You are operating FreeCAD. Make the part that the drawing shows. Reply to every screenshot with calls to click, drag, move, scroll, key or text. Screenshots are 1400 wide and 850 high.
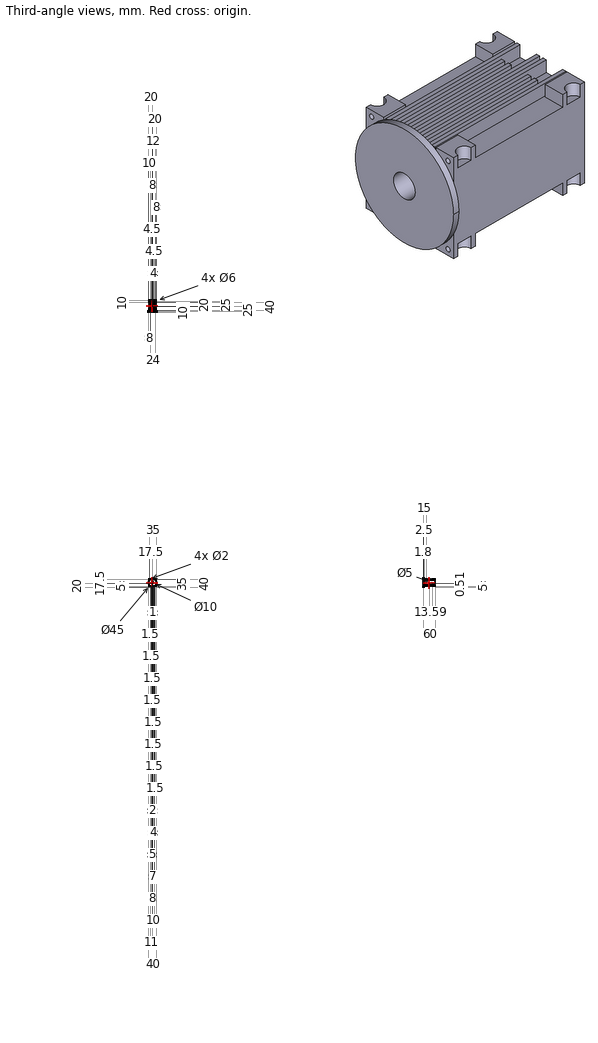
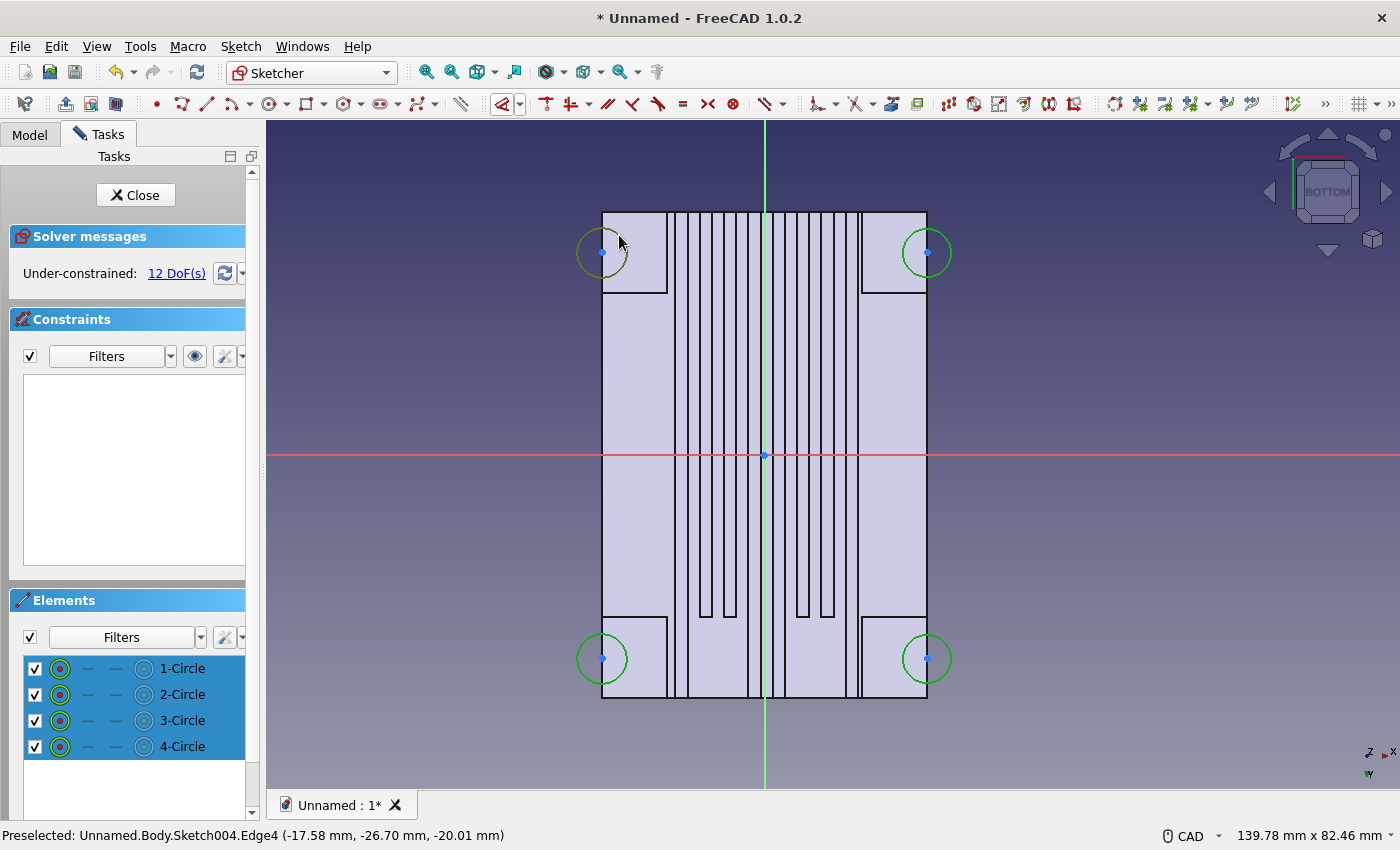
key(e)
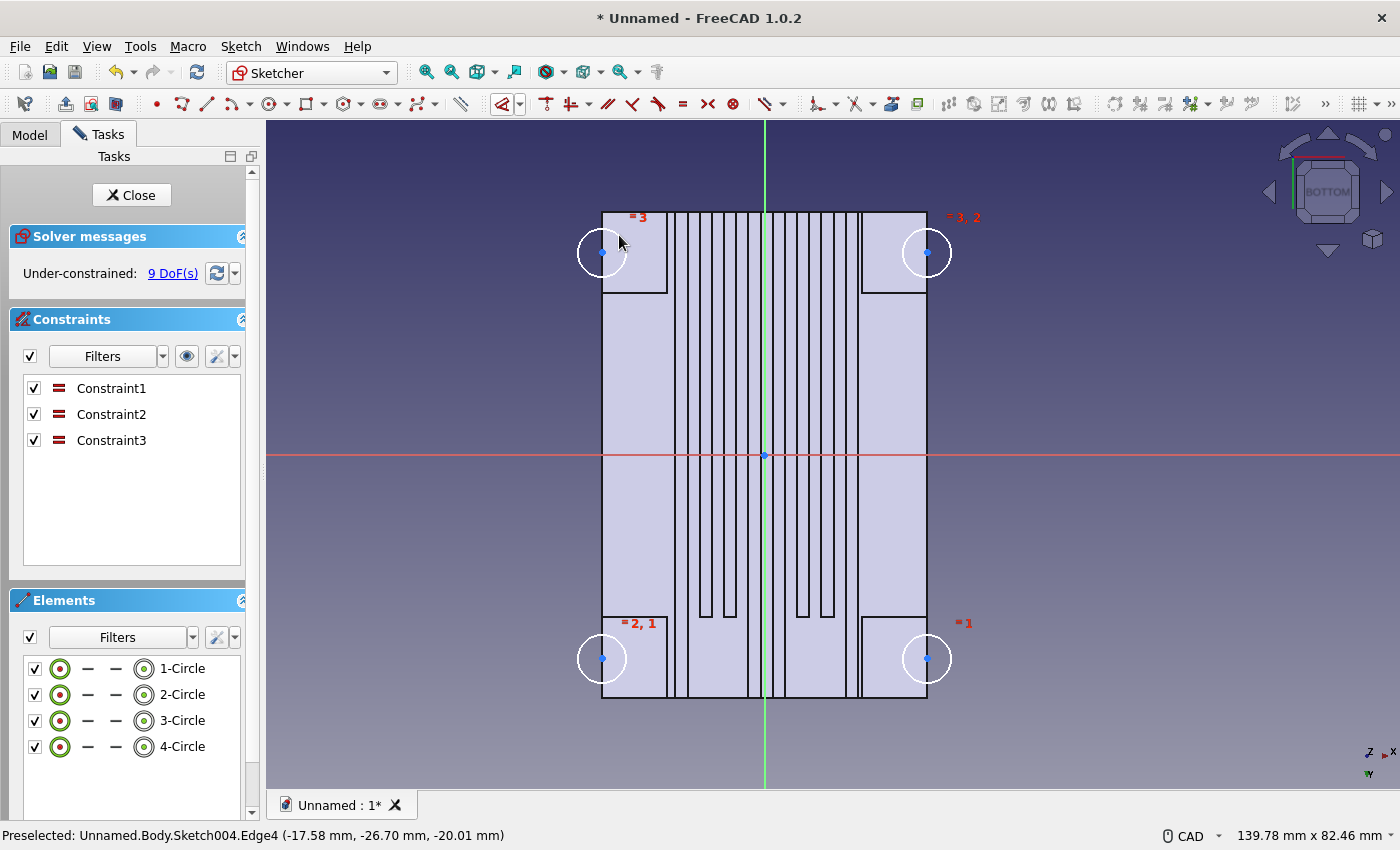
click(927, 659)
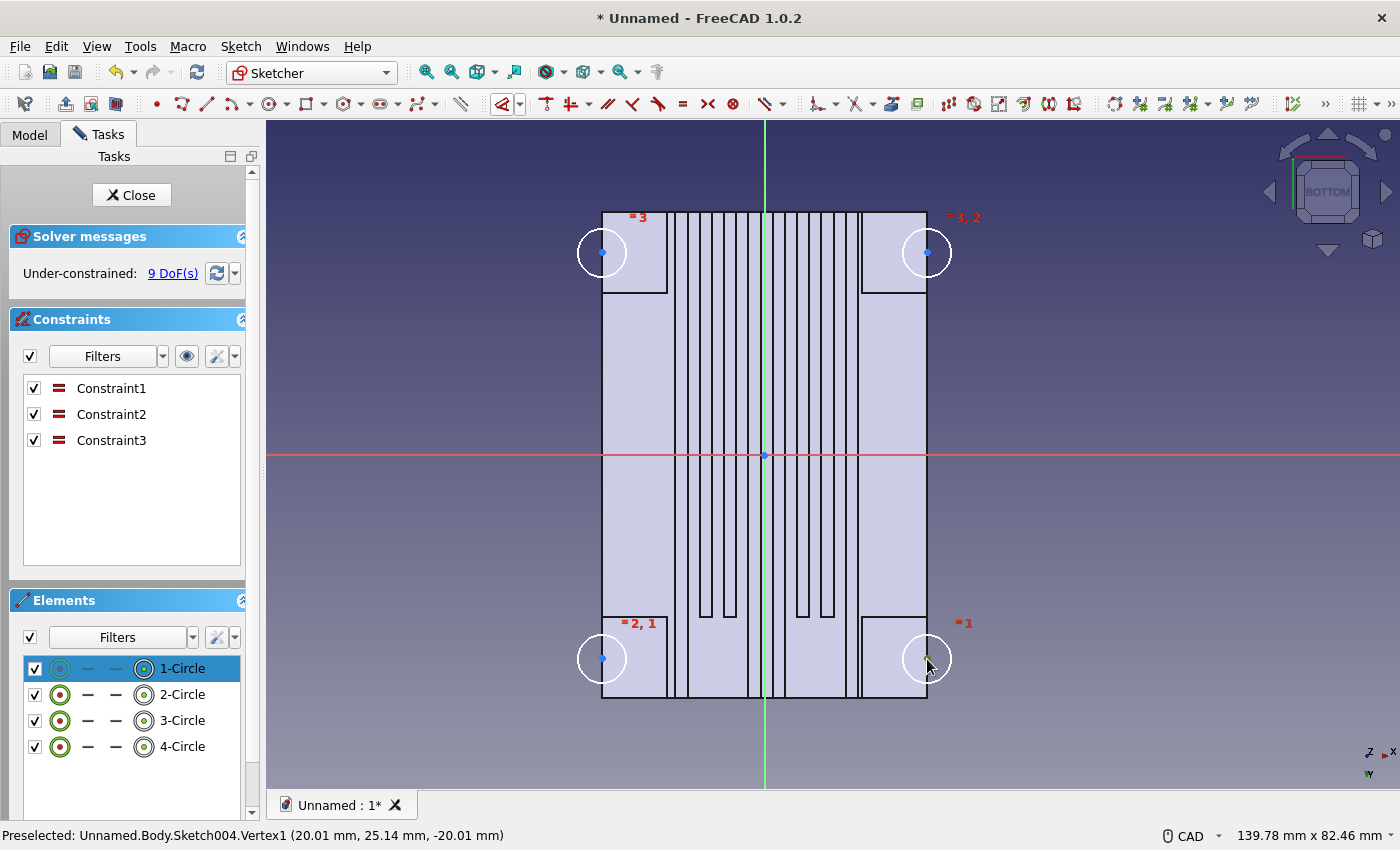
click(602, 659)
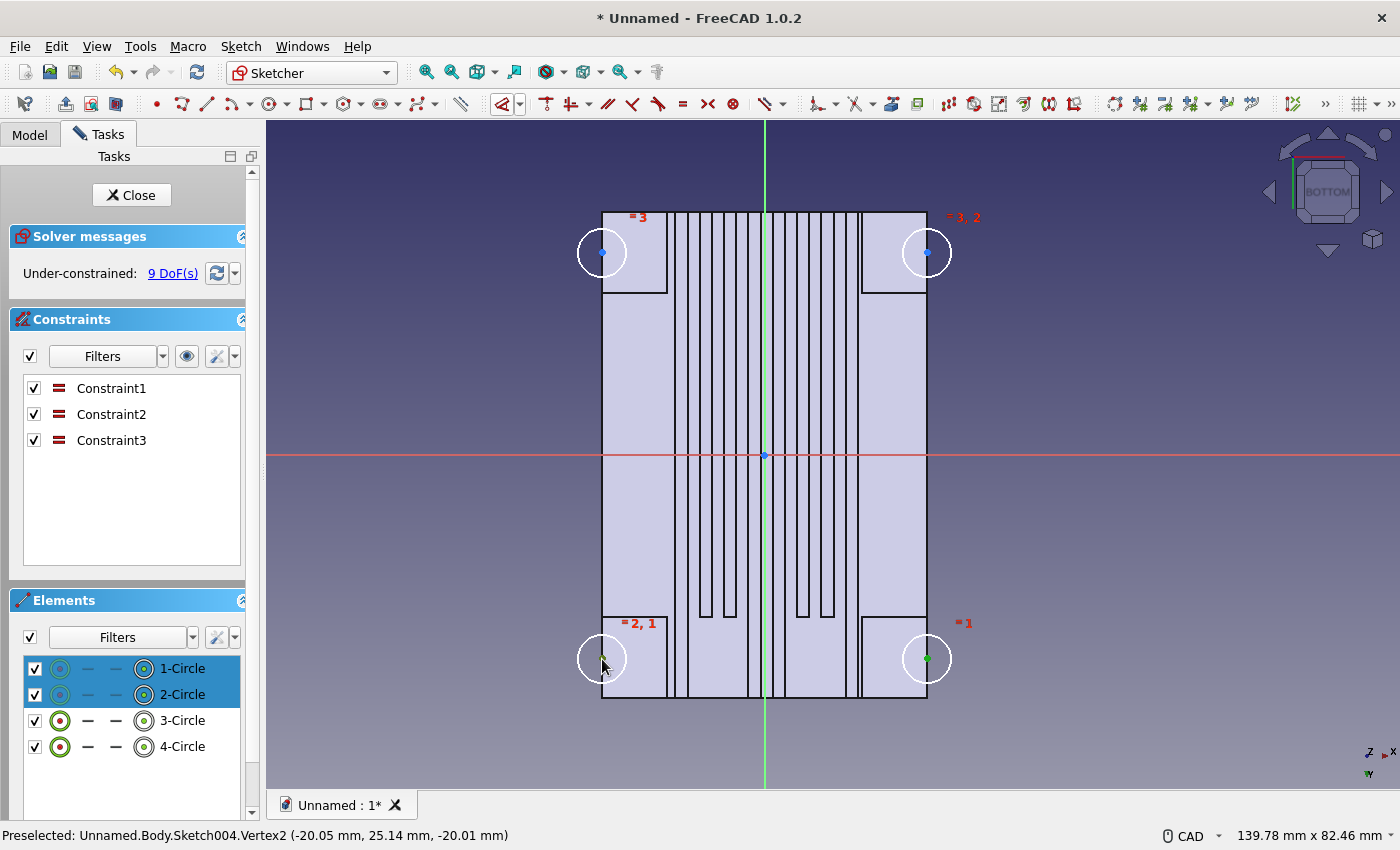
click(588, 104)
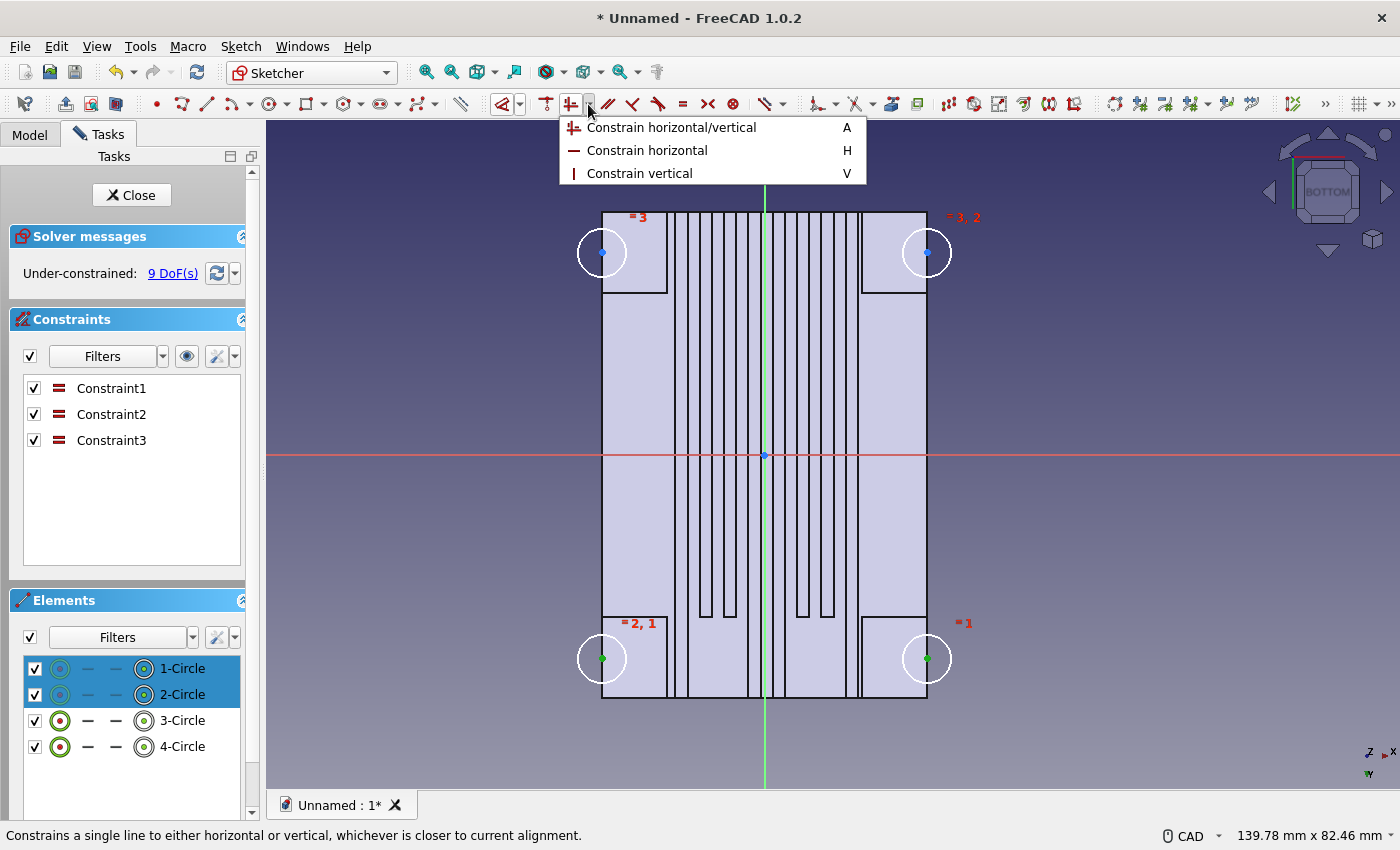
click(713, 150)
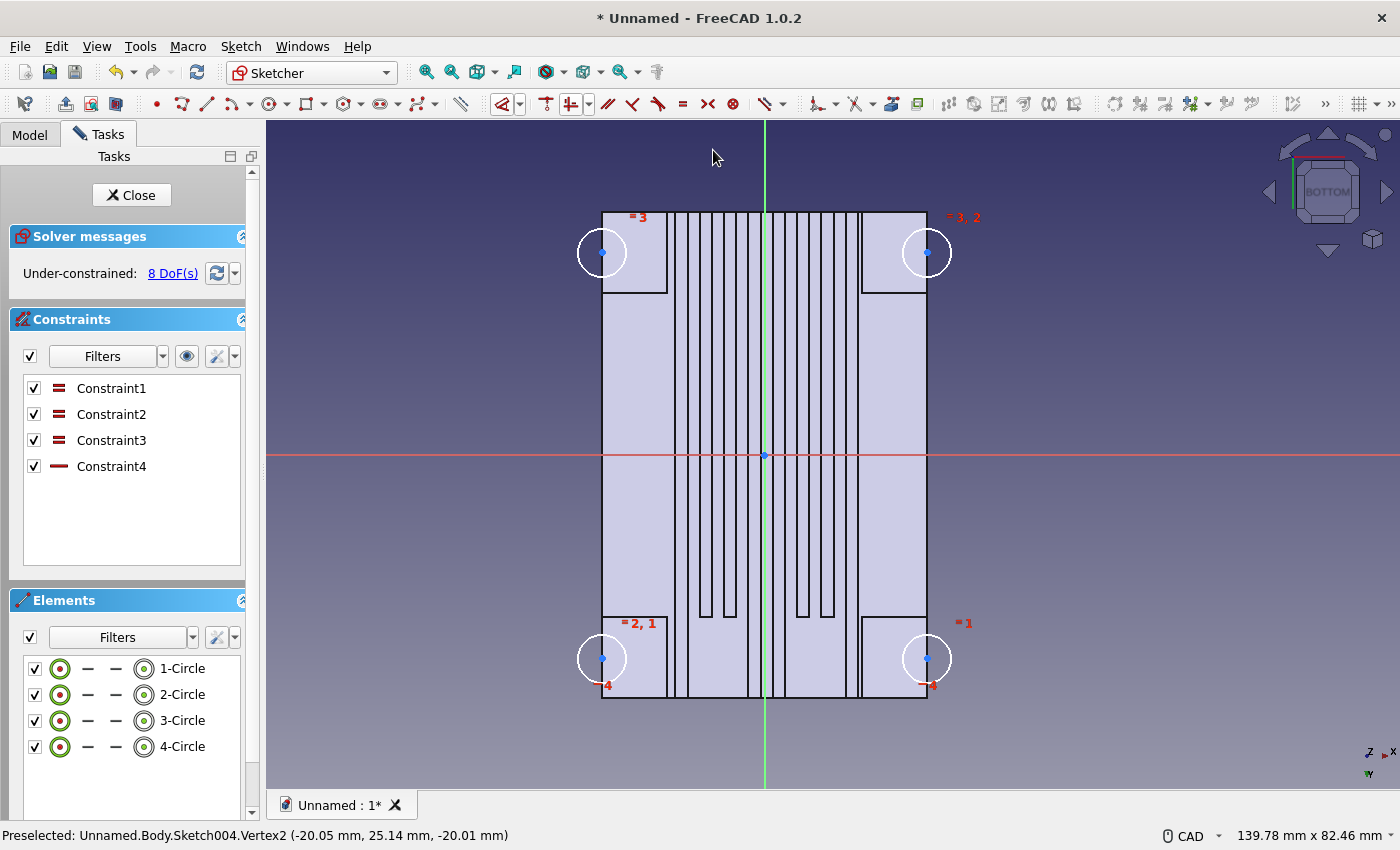
click(927, 659)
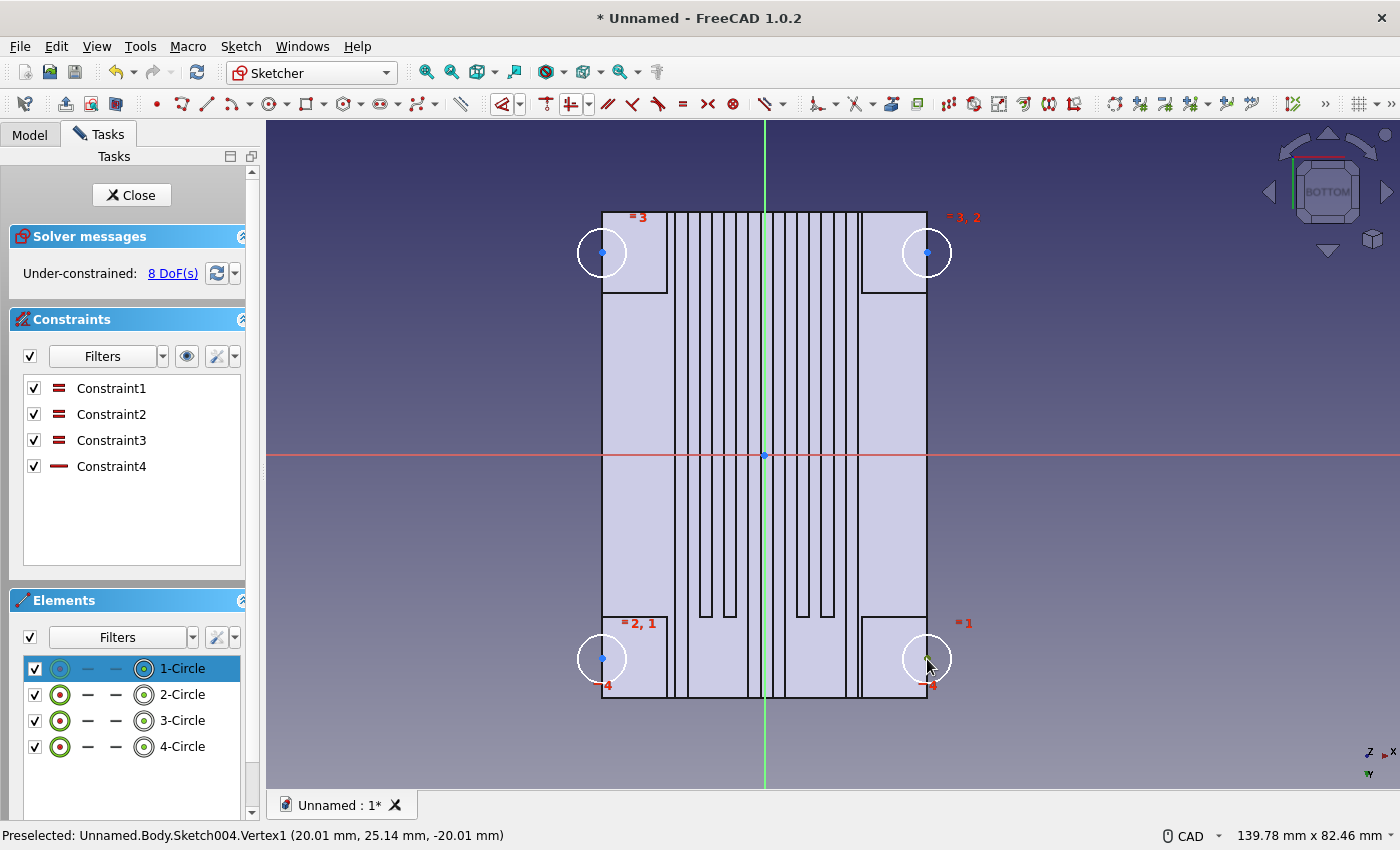
click(927, 253)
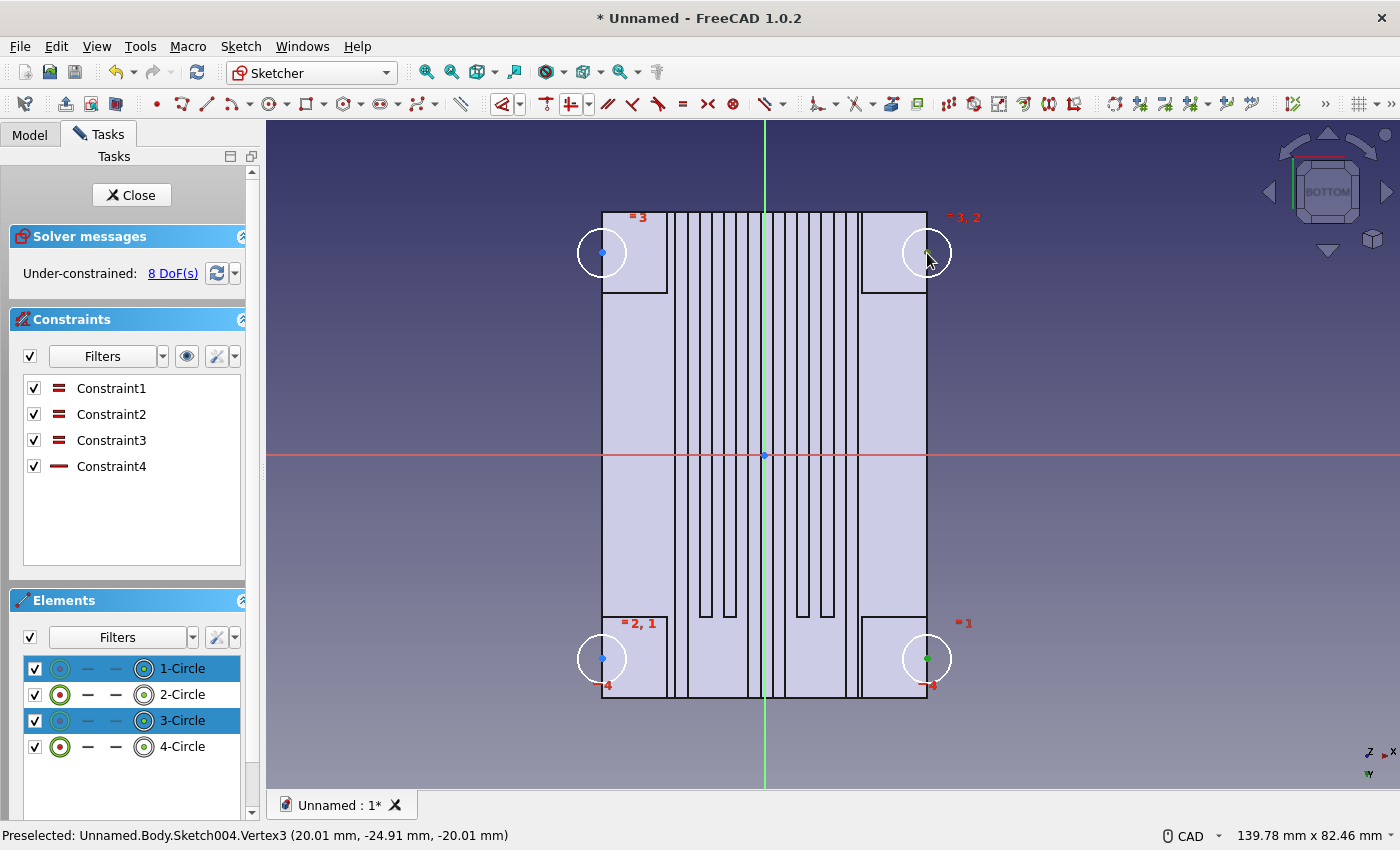
click(588, 104)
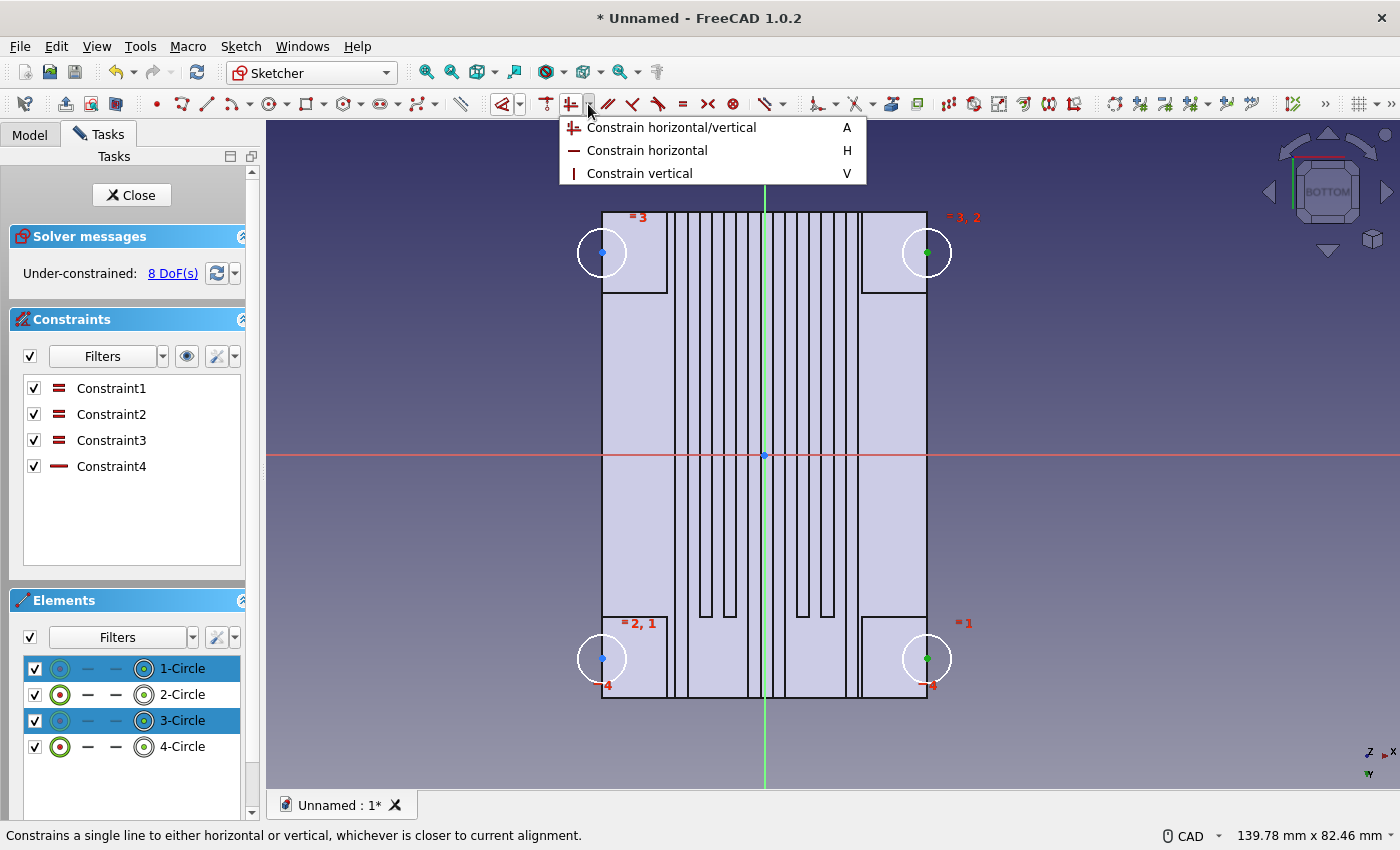
click(713, 174)